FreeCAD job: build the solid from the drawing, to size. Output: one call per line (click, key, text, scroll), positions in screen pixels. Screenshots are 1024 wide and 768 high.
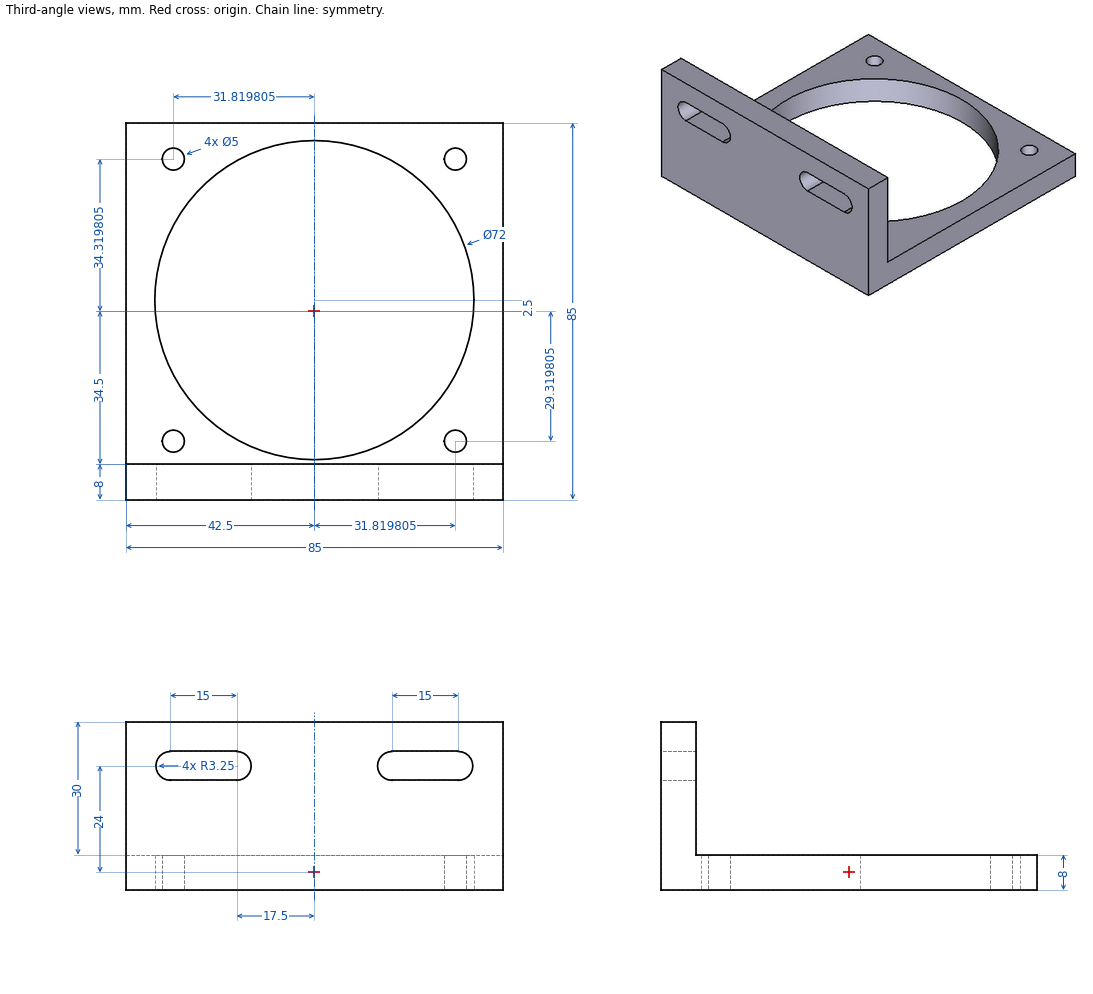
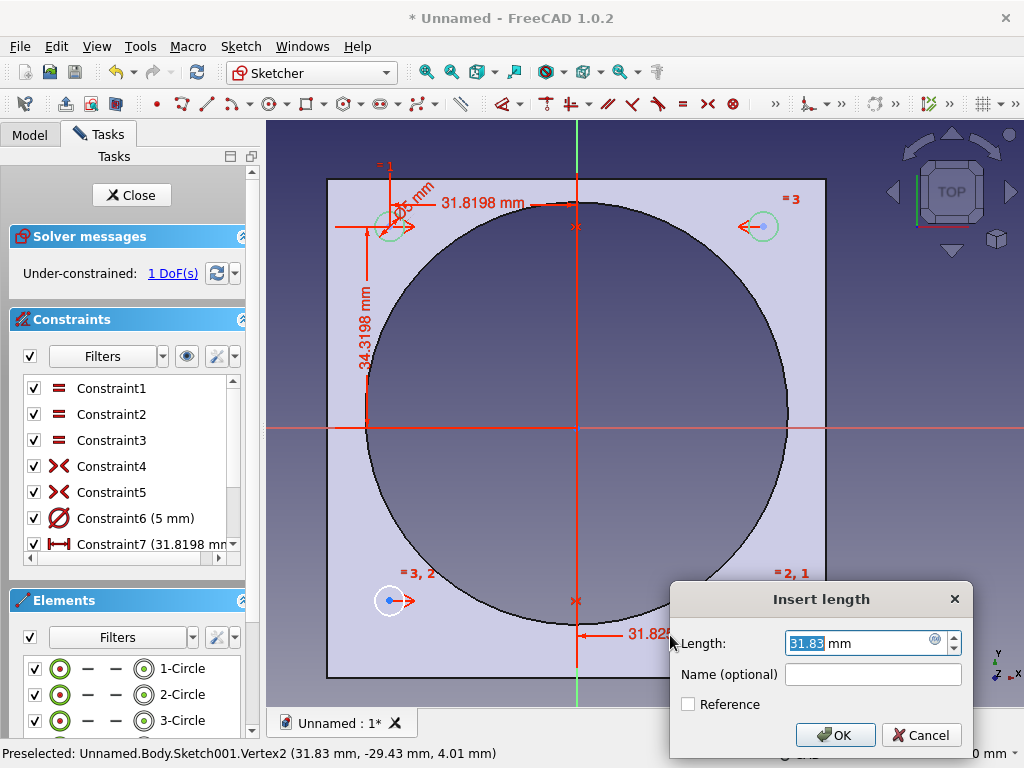
text(31.819805)
key(Return)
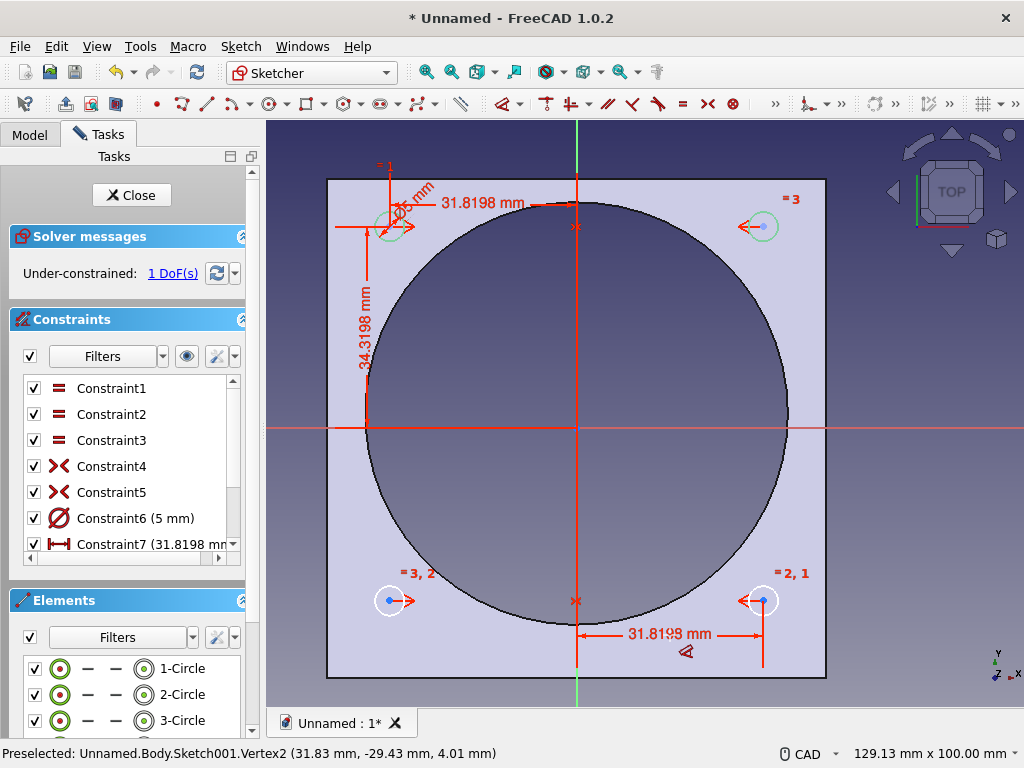
click(763, 601)
click(797, 515)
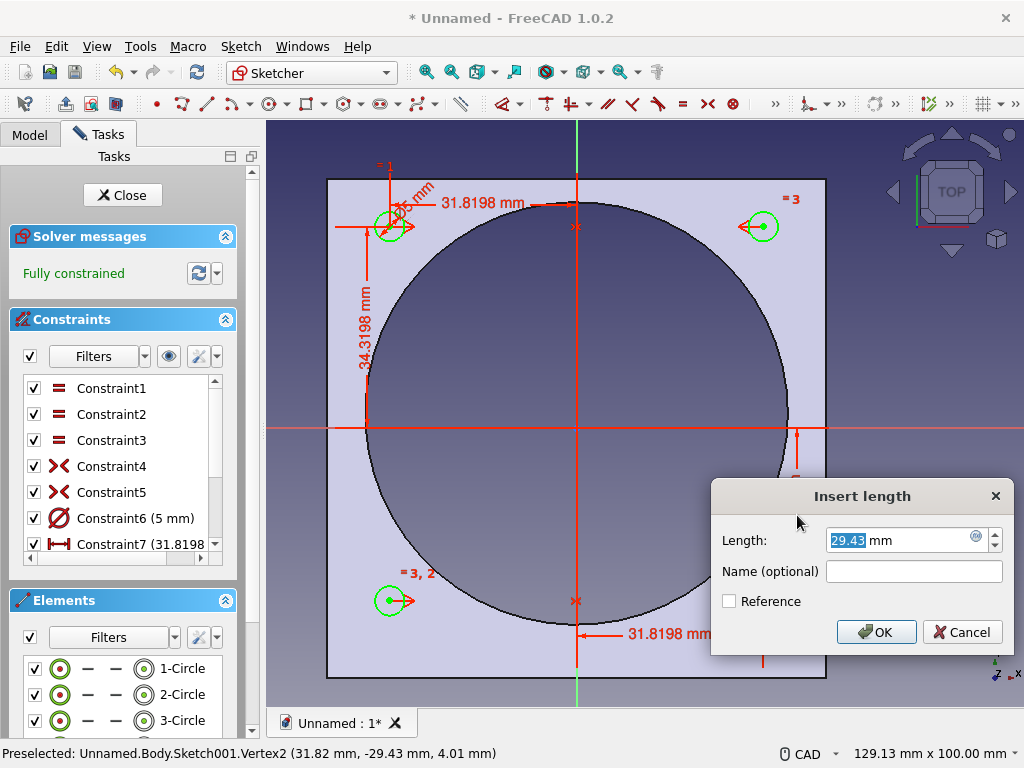
text(29.319805)
key(Return)
key(Escape)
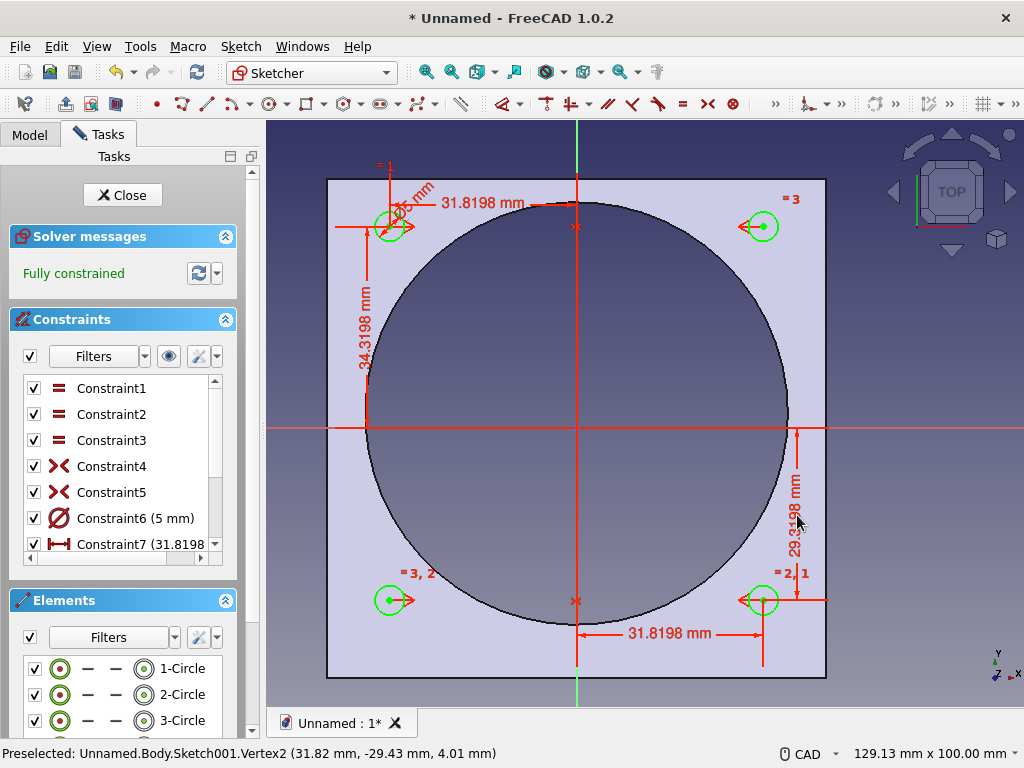
click(123, 195)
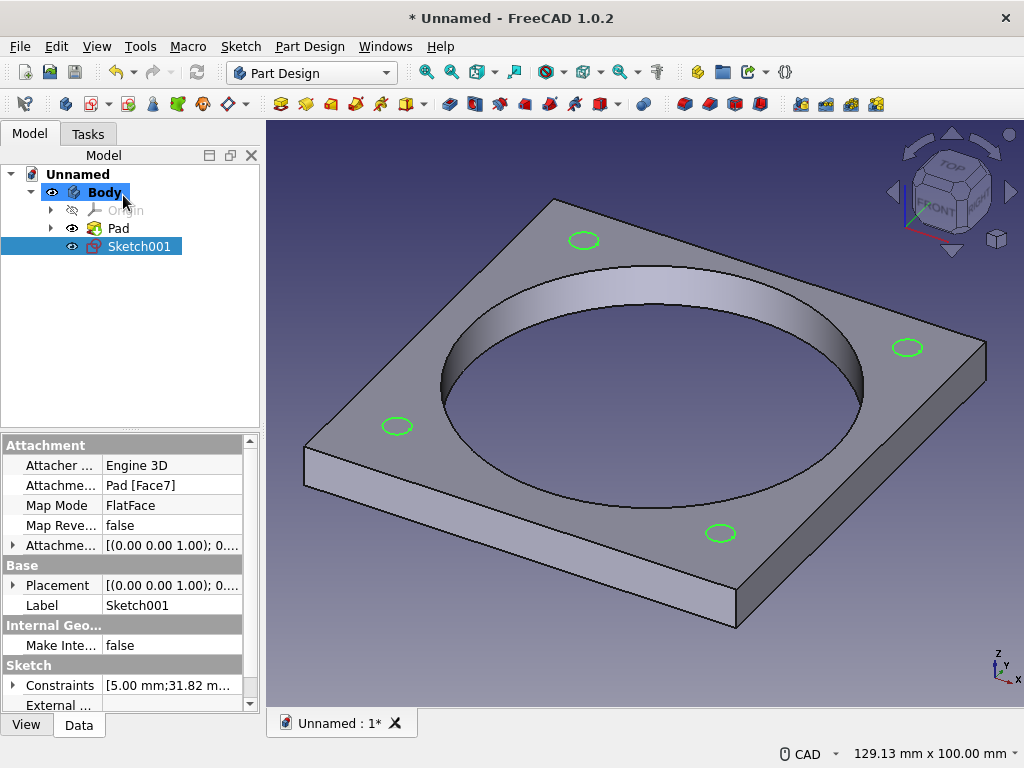
click(450, 104)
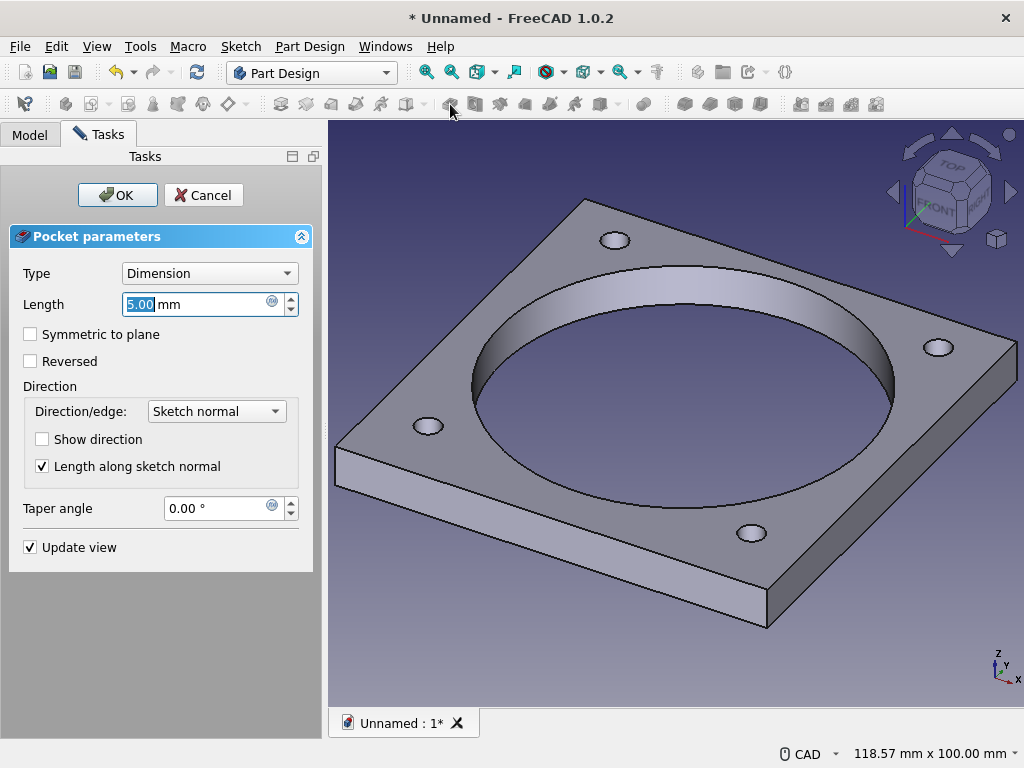
click(210, 274)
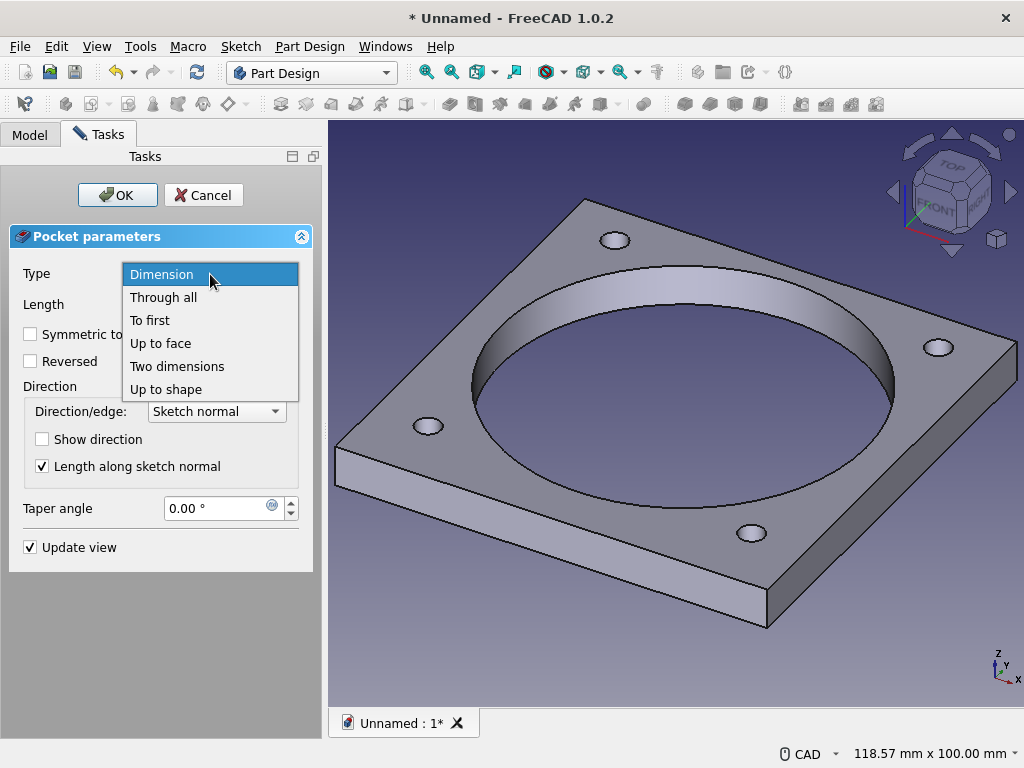
click(208, 298)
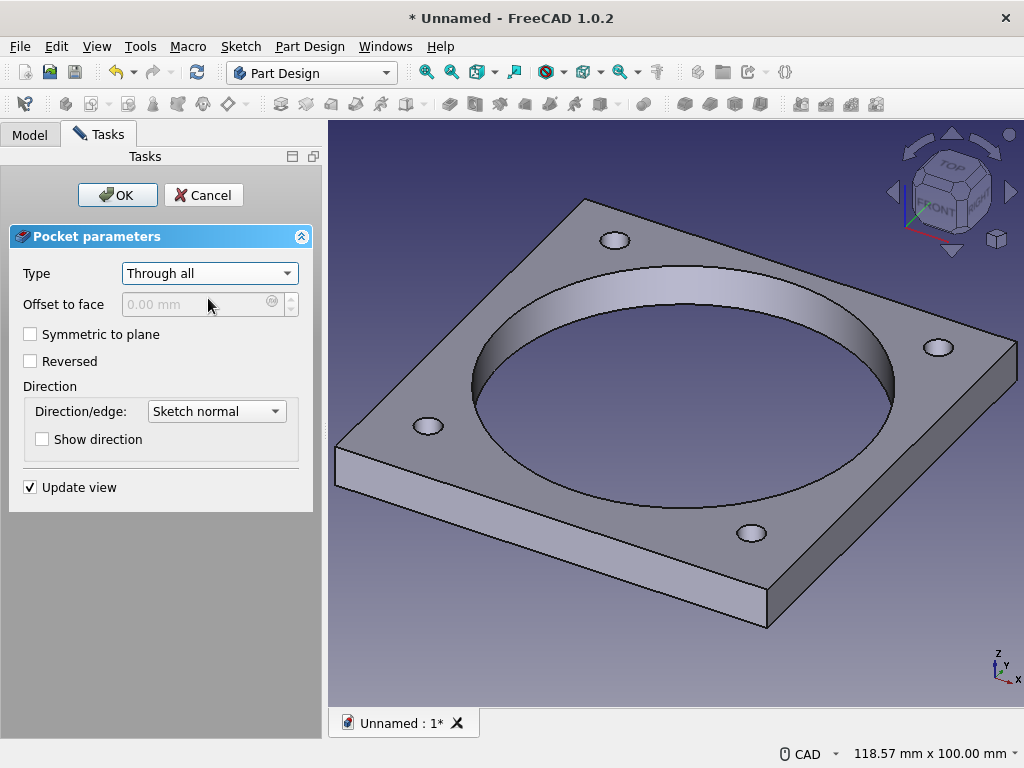
click(118, 195)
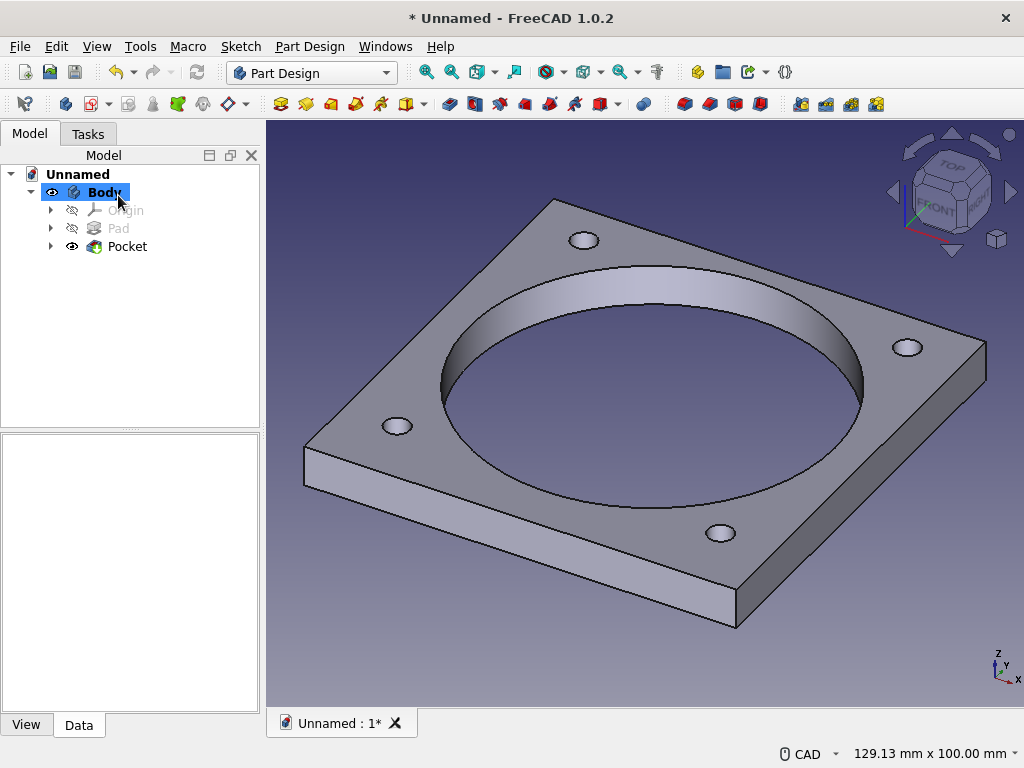
click(901, 384)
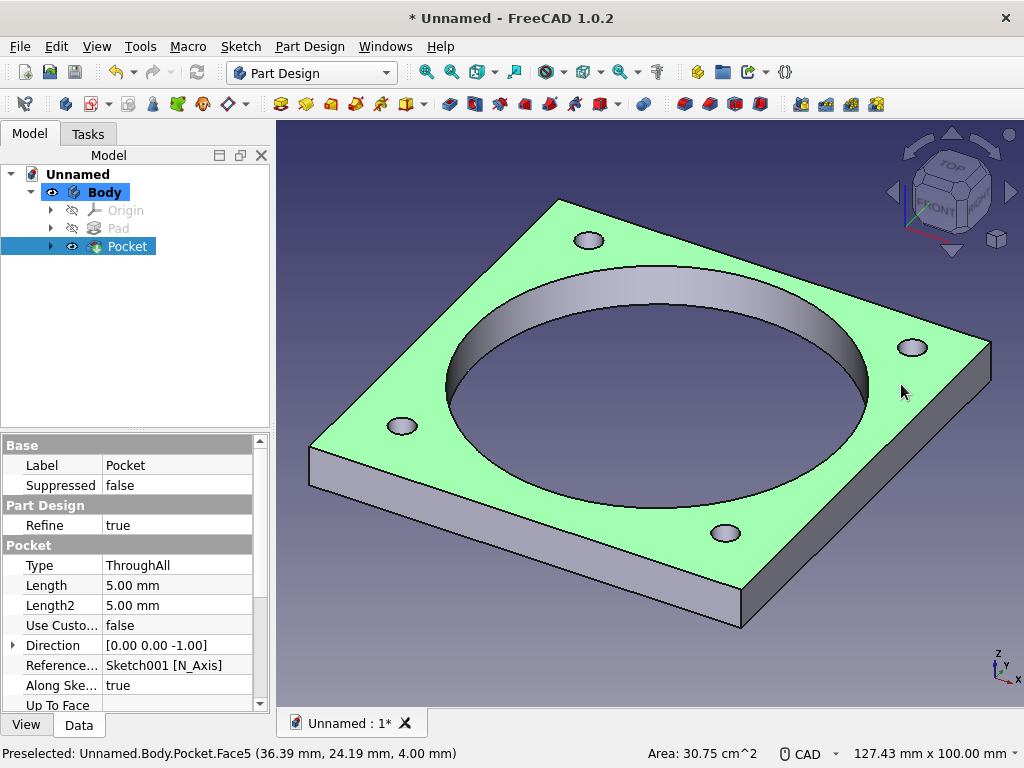
click(90, 104)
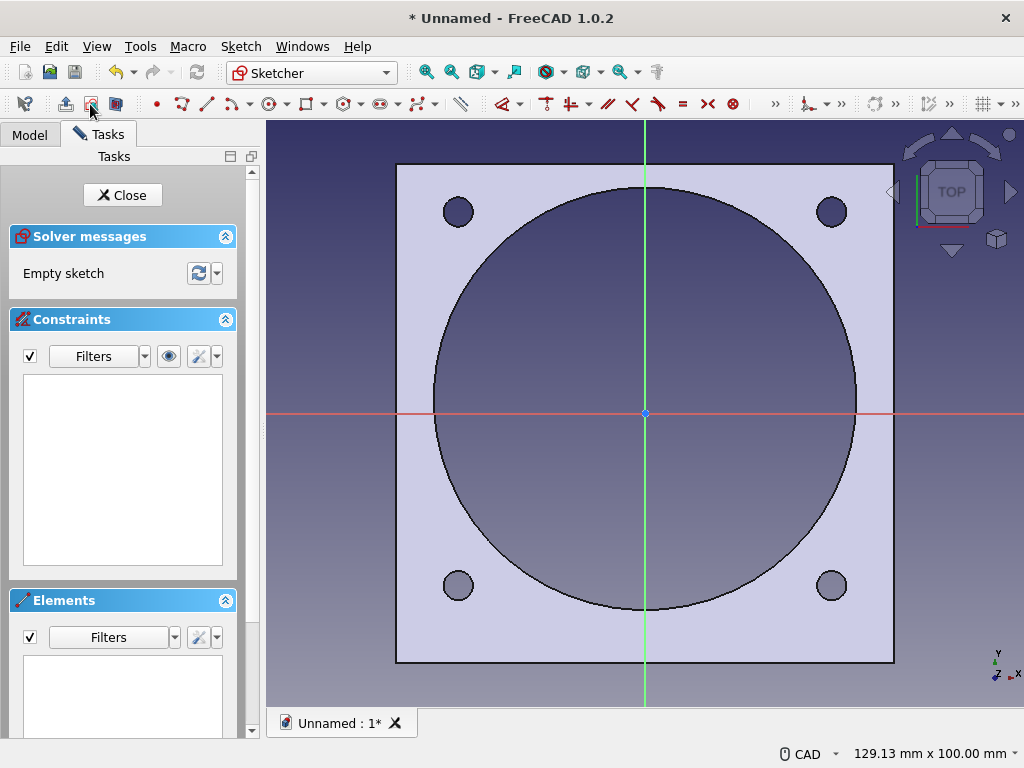
scroll(294, 148, down, 1)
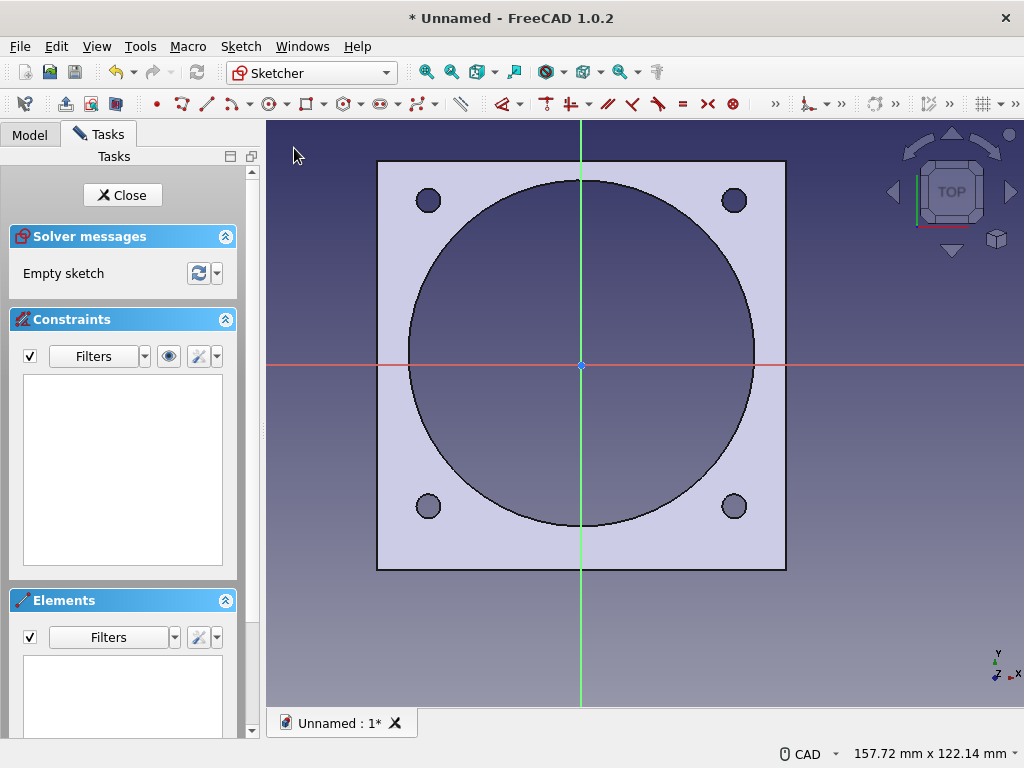
key(g)
key(r)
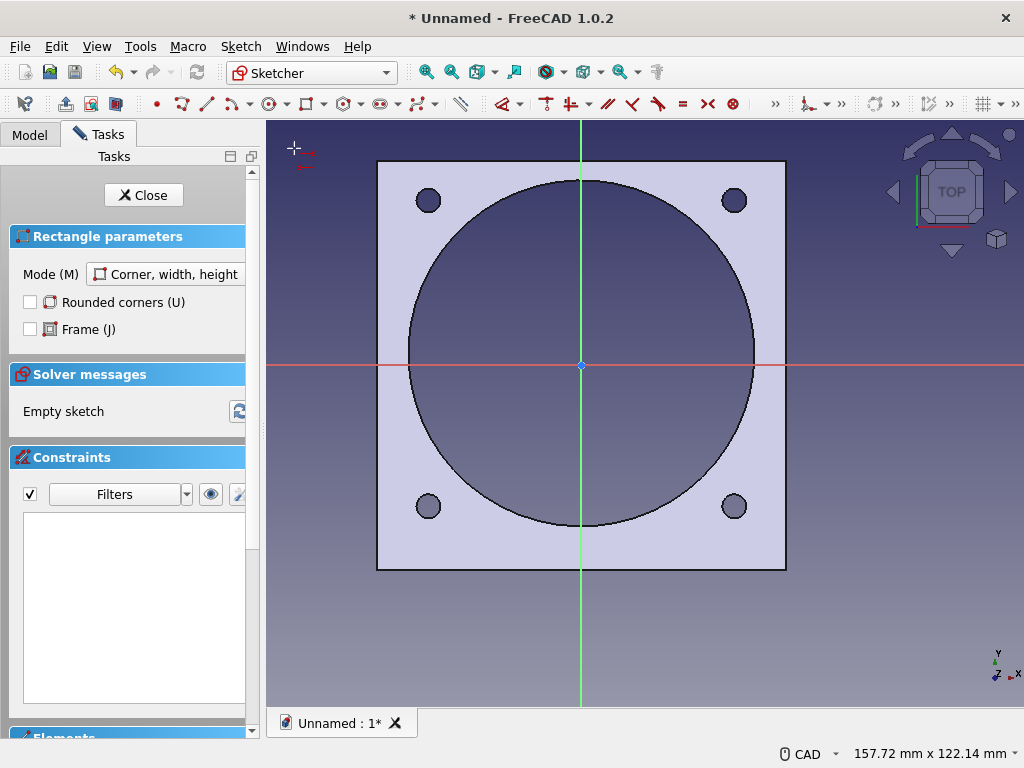
click(377, 531)
click(786, 570)
key(Escape)